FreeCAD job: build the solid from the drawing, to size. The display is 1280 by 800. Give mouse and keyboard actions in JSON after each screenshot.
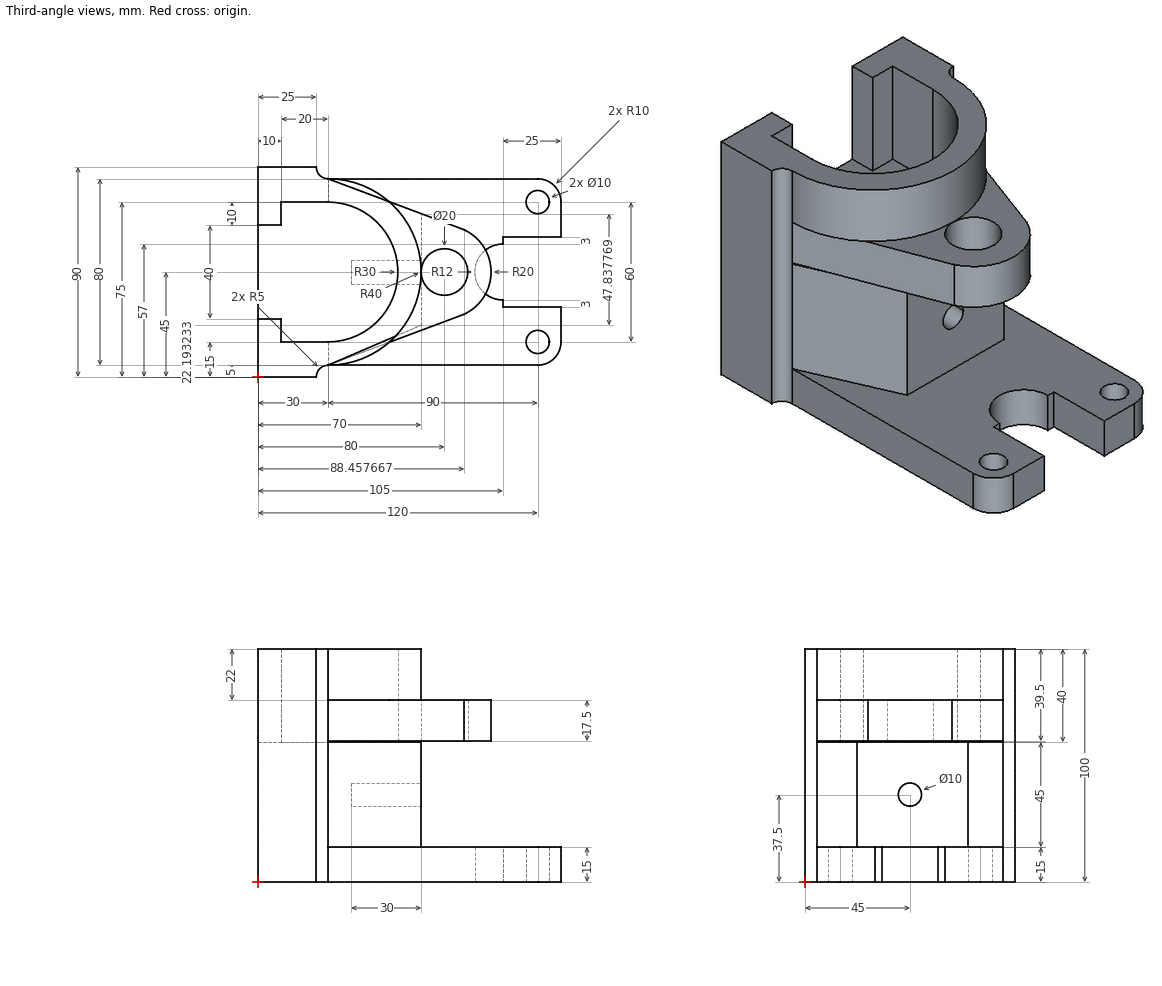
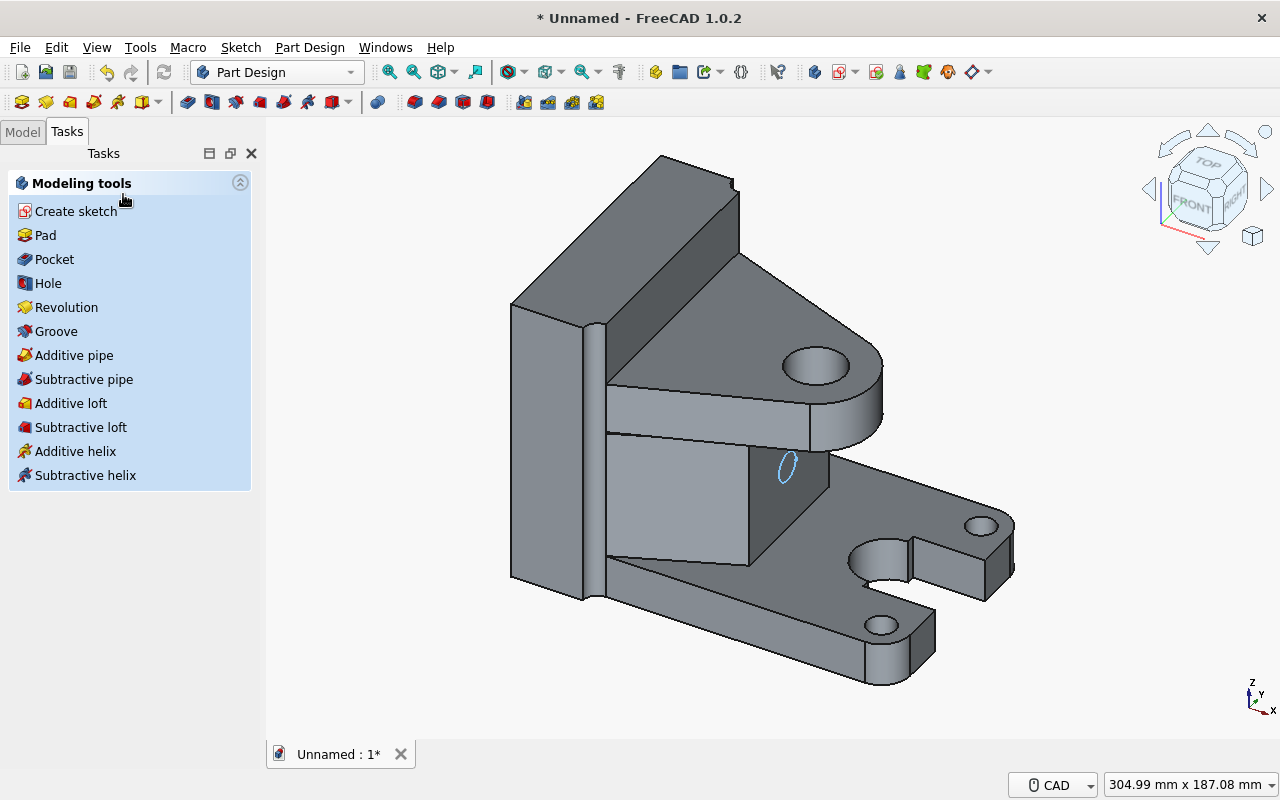
{"action": "left_click", "coordinate": [188, 102]}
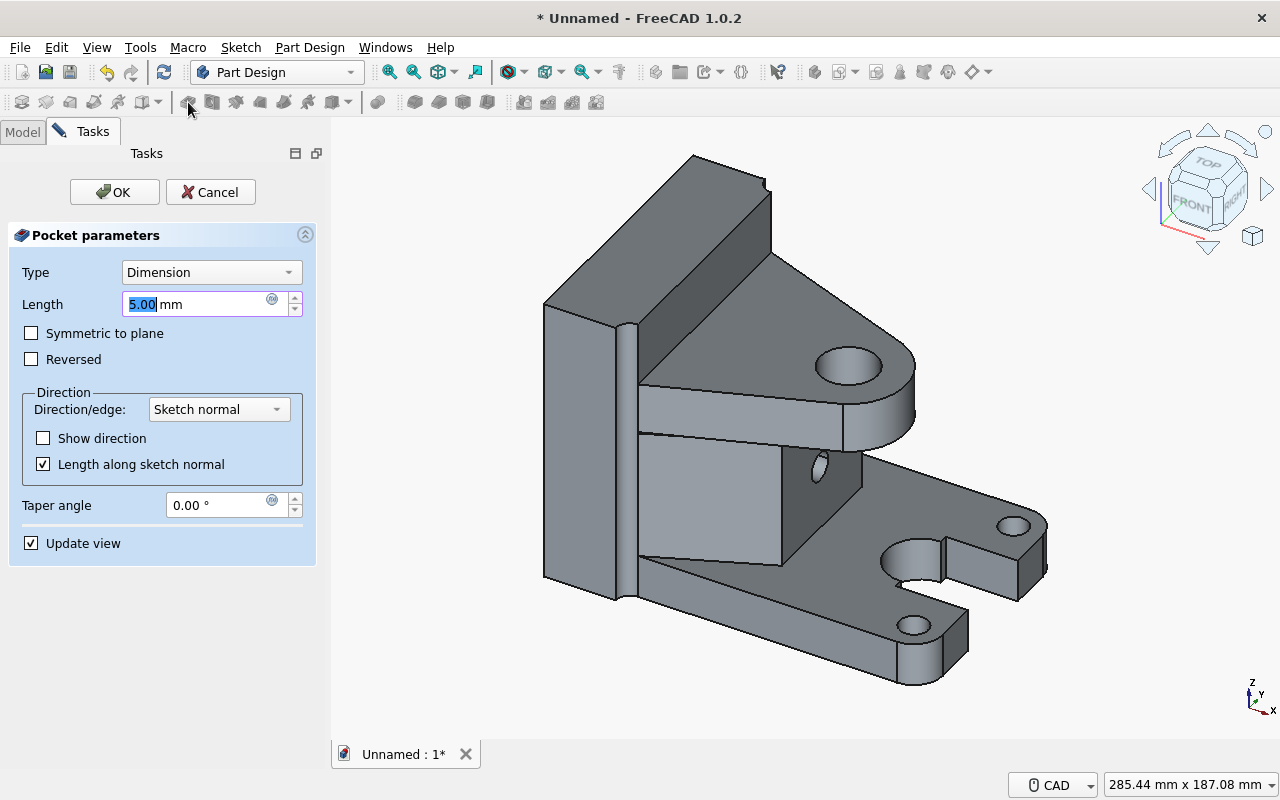
{"action": "type", "text": "30"}
{"action": "key", "text": "Tab"}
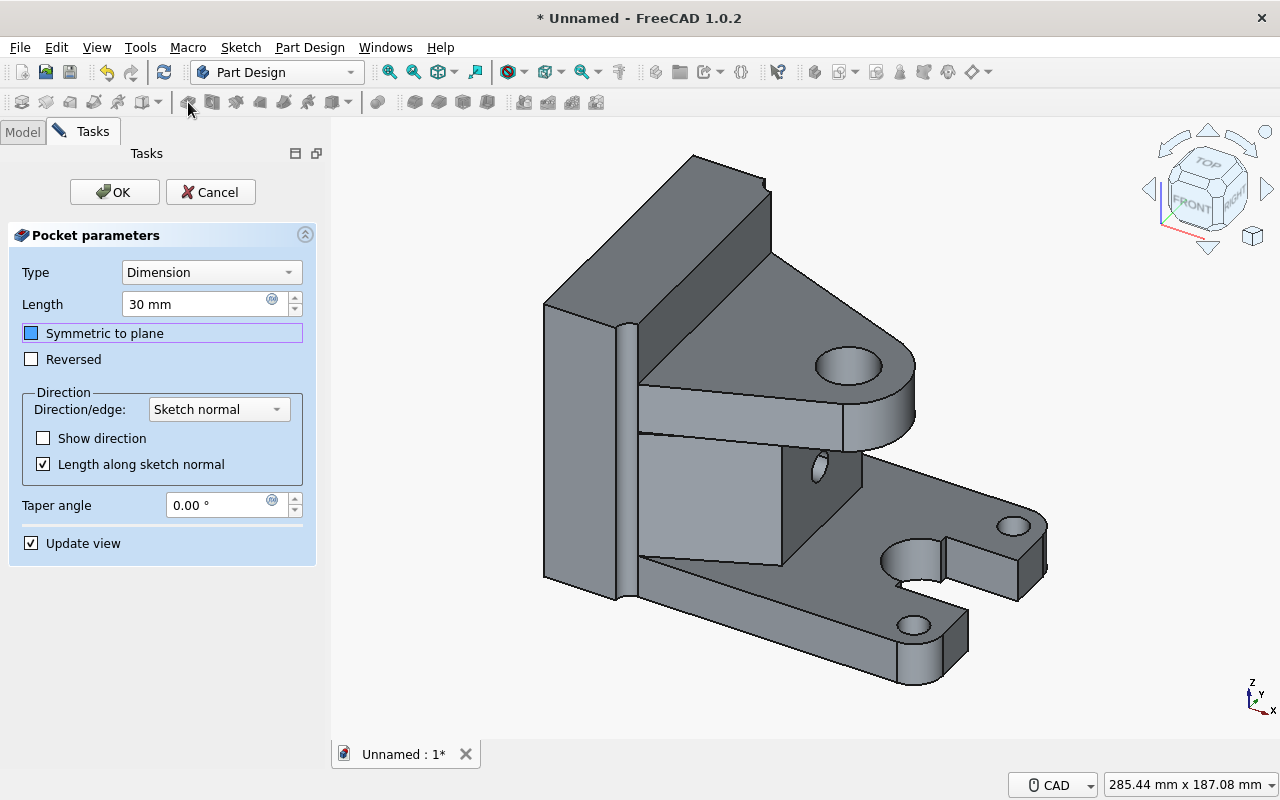
{"action": "left_click", "coordinate": [115, 192]}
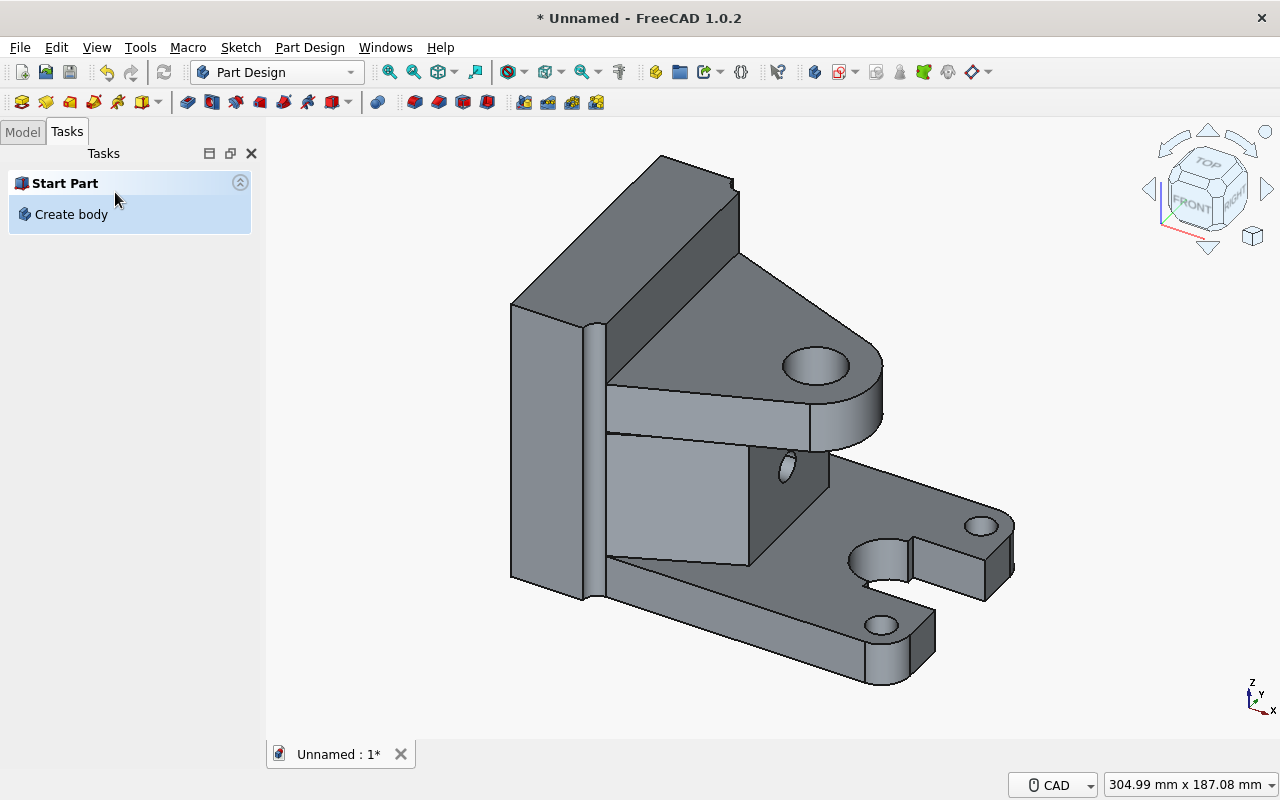
{"action": "left_click", "coordinate": [672, 201]}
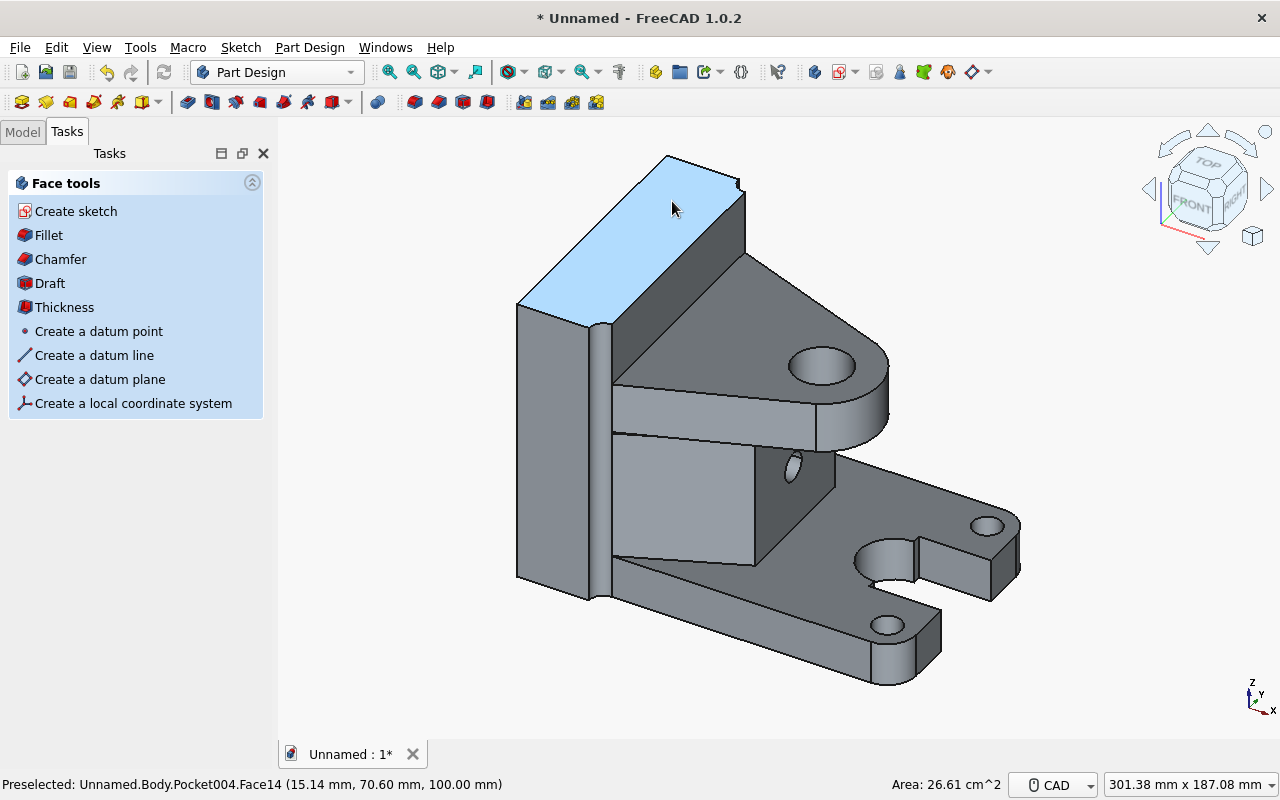
{"action": "left_click", "coordinate": [840, 72]}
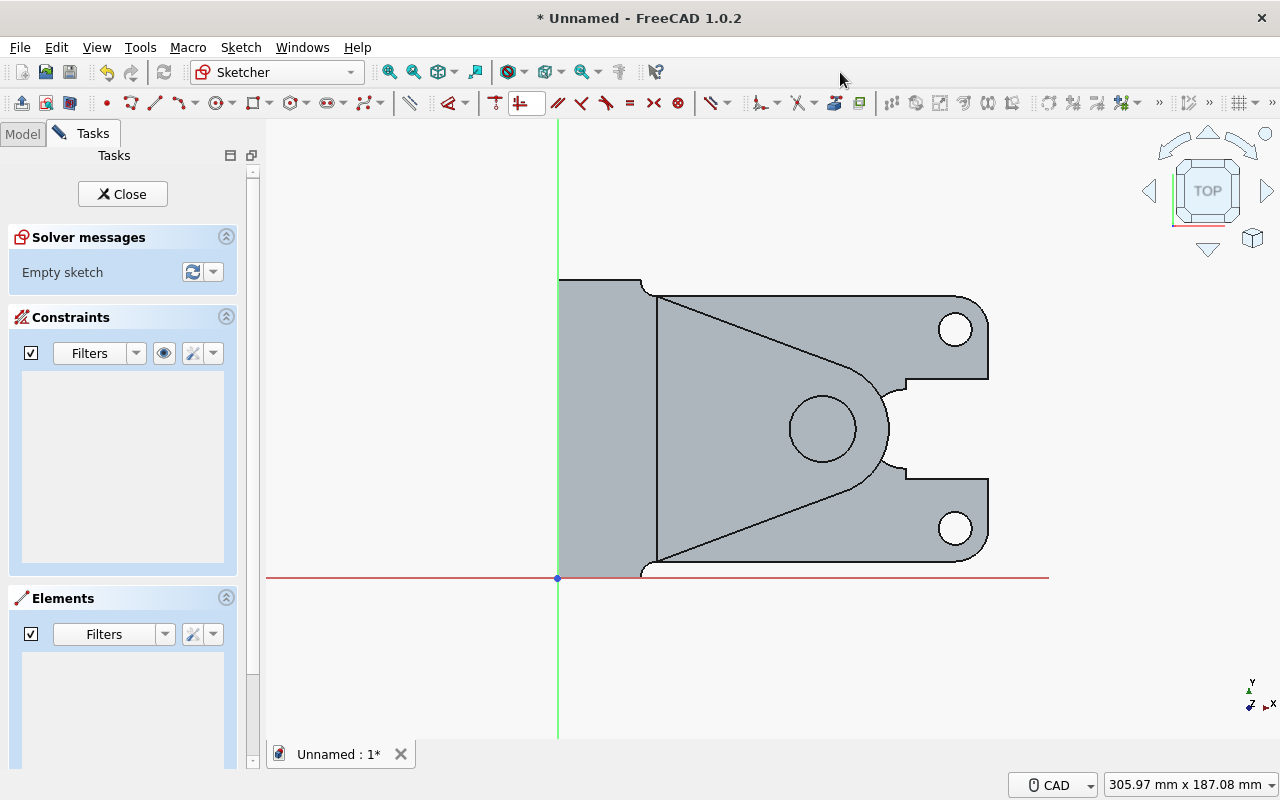
{"action": "scroll", "coordinate": [611, 454], "scroll_direction": "up", "scroll_amount": 2}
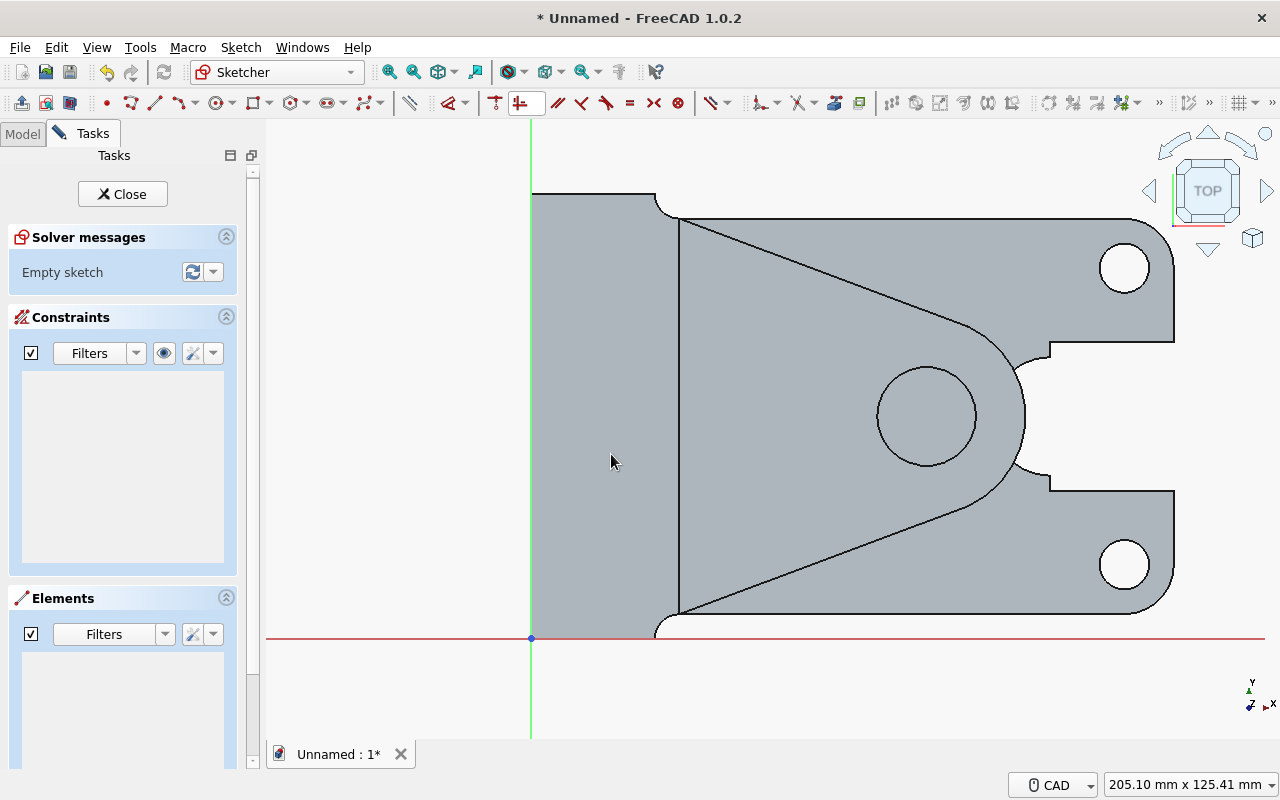
{"action": "left_click", "coordinate": [156, 104]}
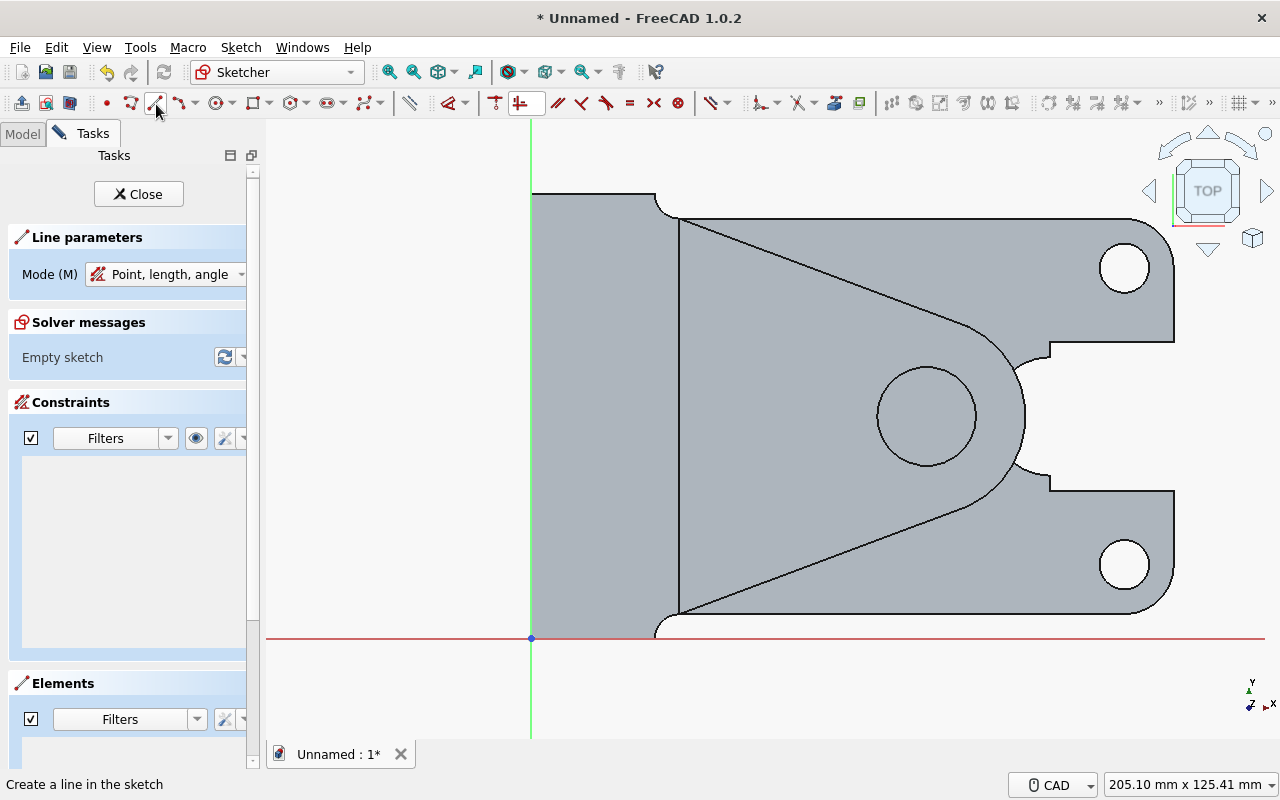
{"action": "left_click", "coordinate": [679, 219]}
{"action": "left_click", "coordinate": [679, 268]}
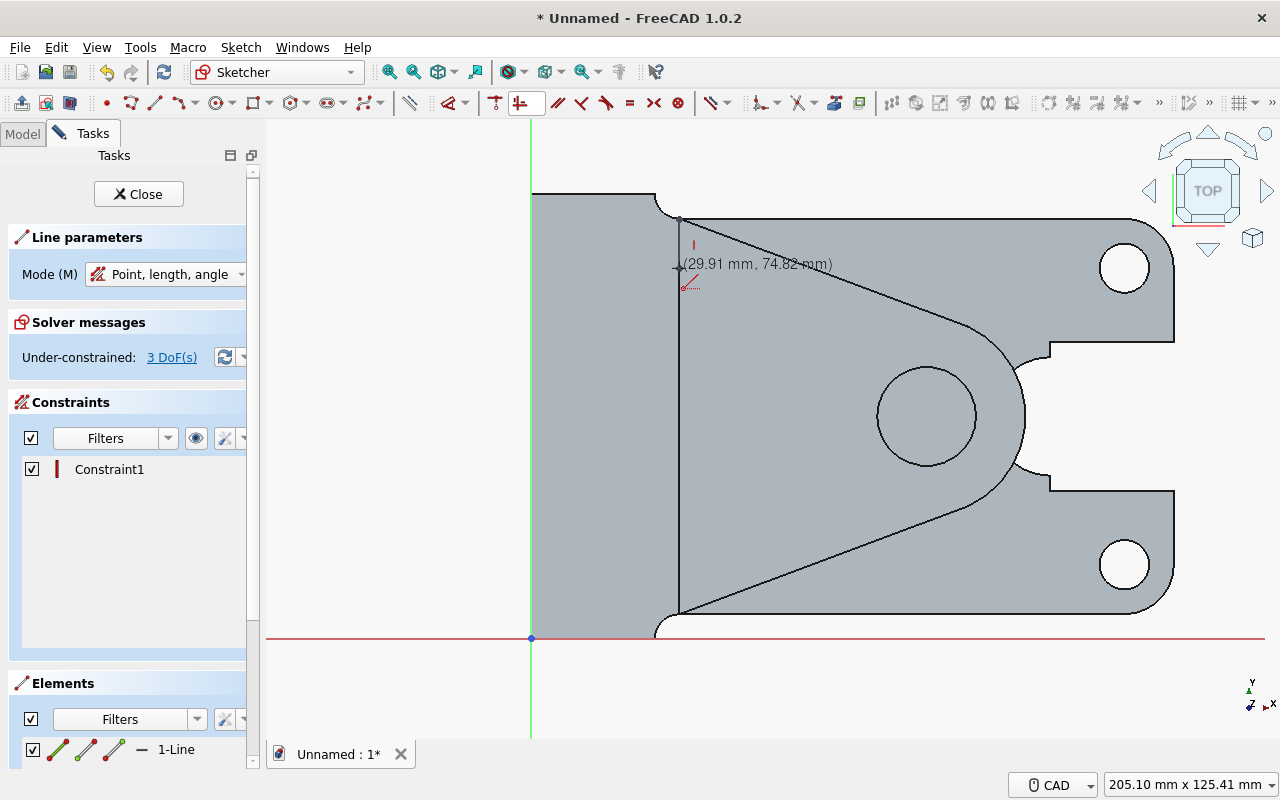
{"action": "left_click", "coordinate": [679, 565]}
{"action": "left_click", "coordinate": [679, 614]}